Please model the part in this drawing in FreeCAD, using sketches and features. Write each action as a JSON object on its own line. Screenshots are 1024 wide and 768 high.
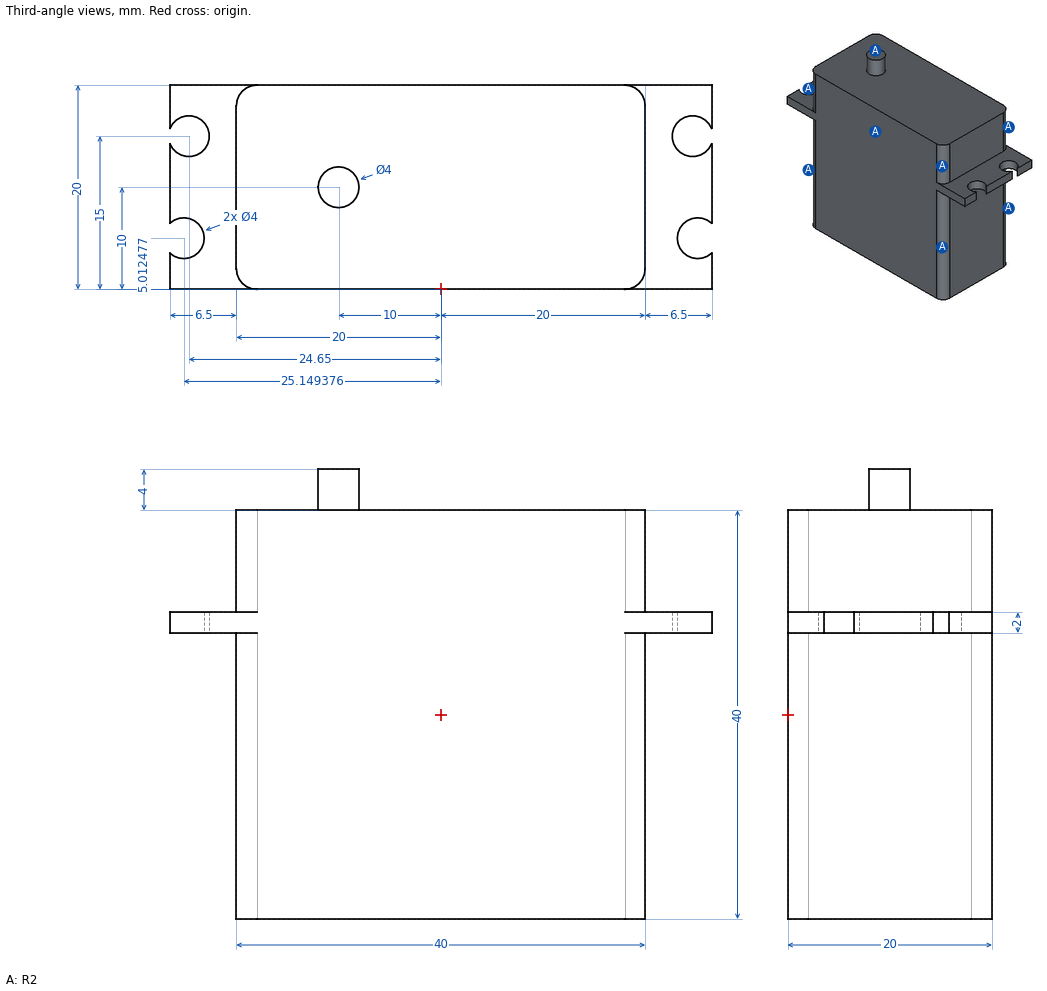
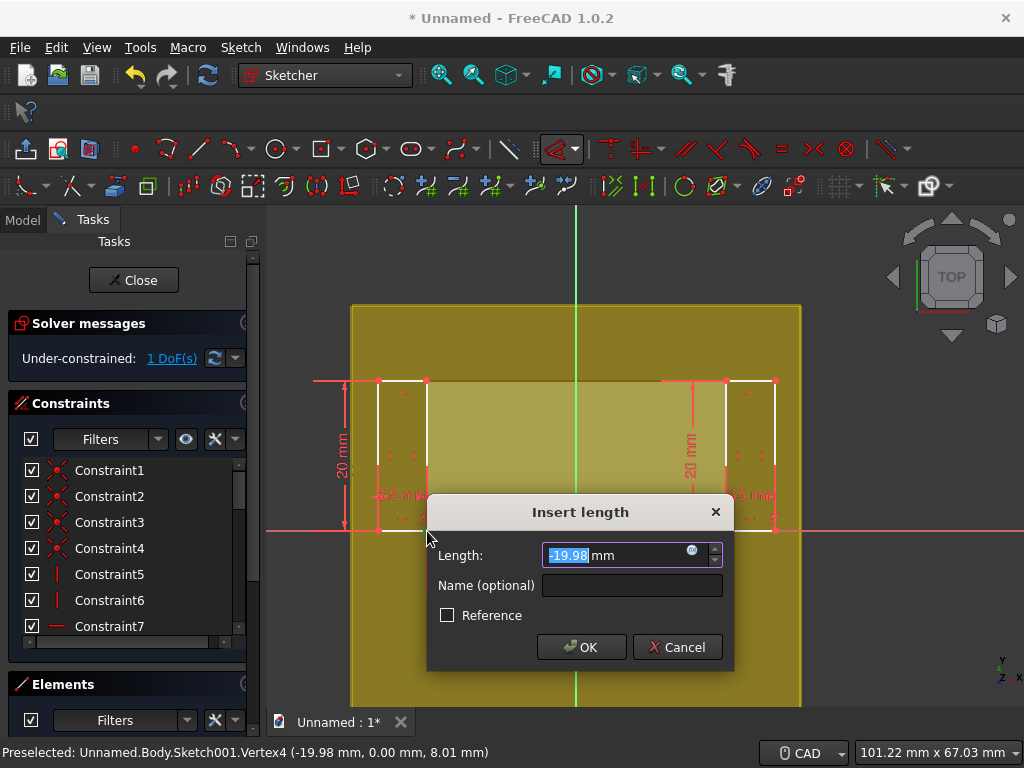
{"action": "type", "text": "-20"}
{"action": "key", "text": "Return"}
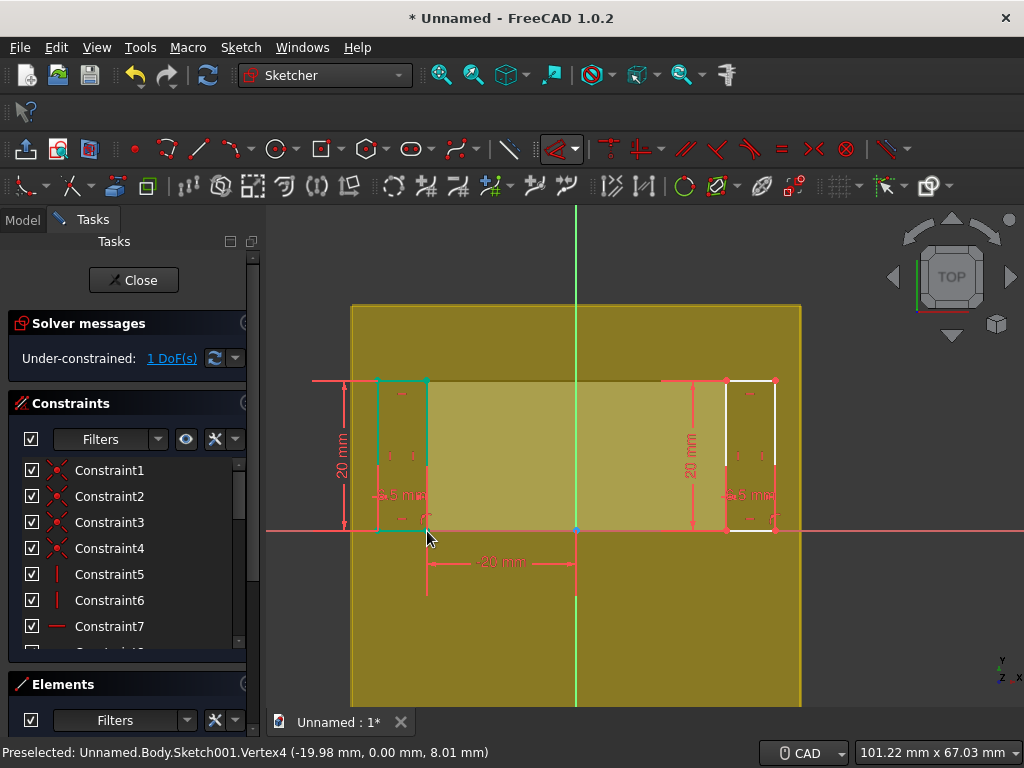
{"action": "left_click", "coordinate": [726, 381]}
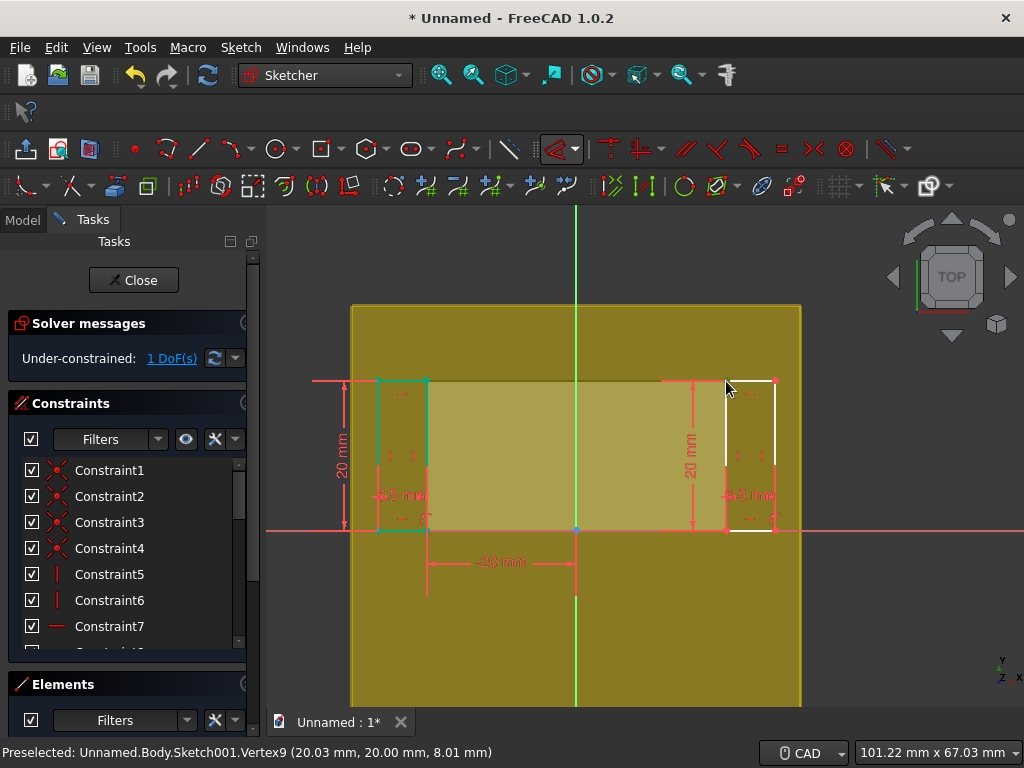
{"action": "key", "text": "l"}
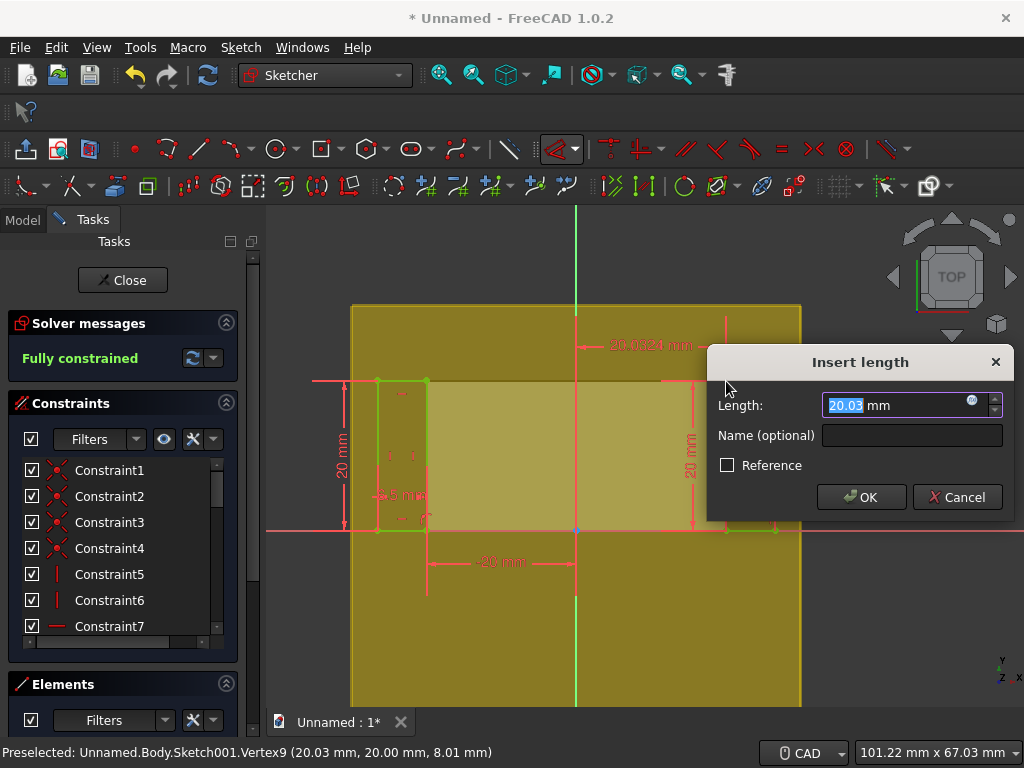
{"action": "type", "text": "20"}
{"action": "key", "text": "Return"}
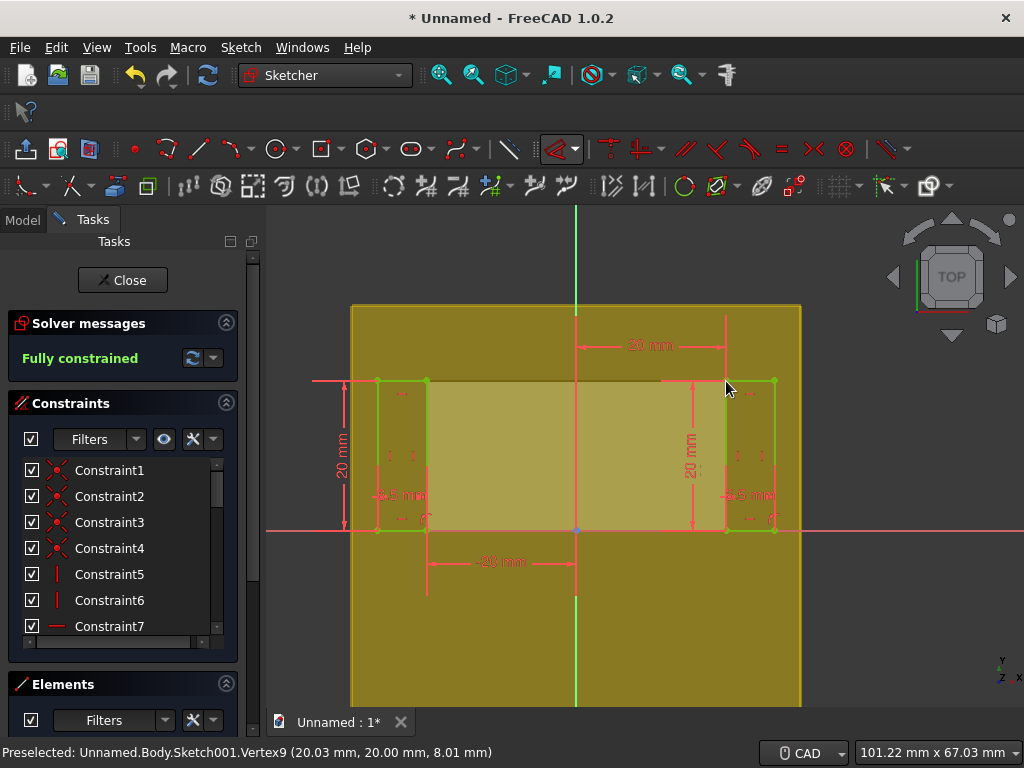
{"action": "left_click", "coordinate": [123, 280]}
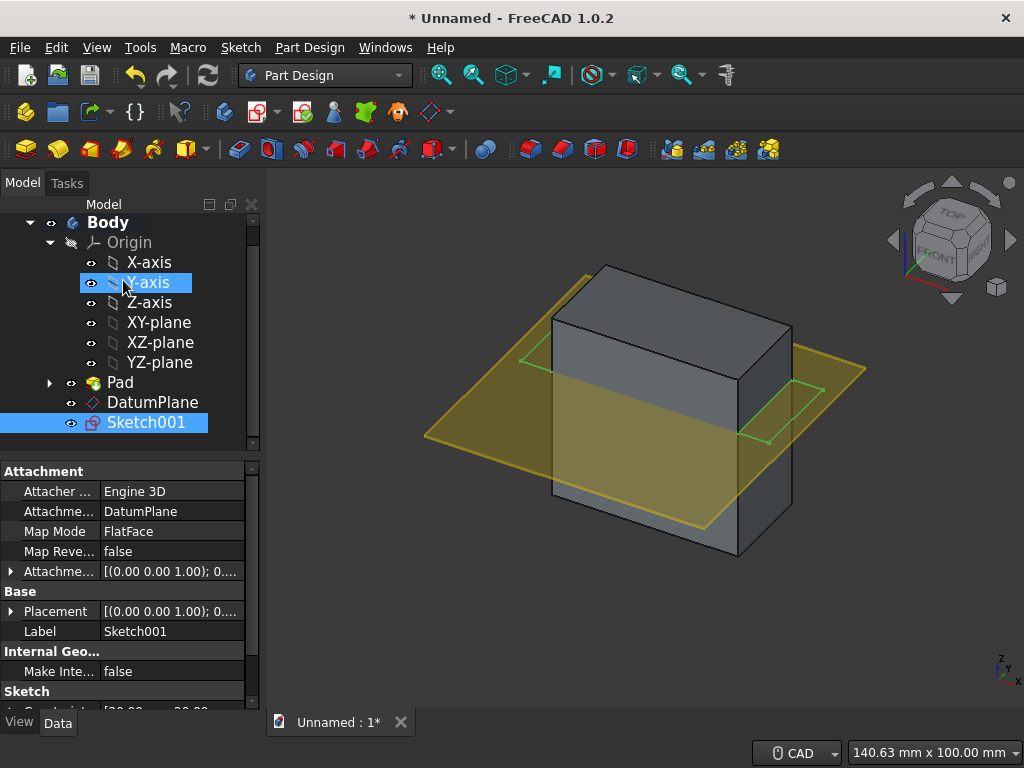
{"action": "left_click", "coordinate": [26, 150]}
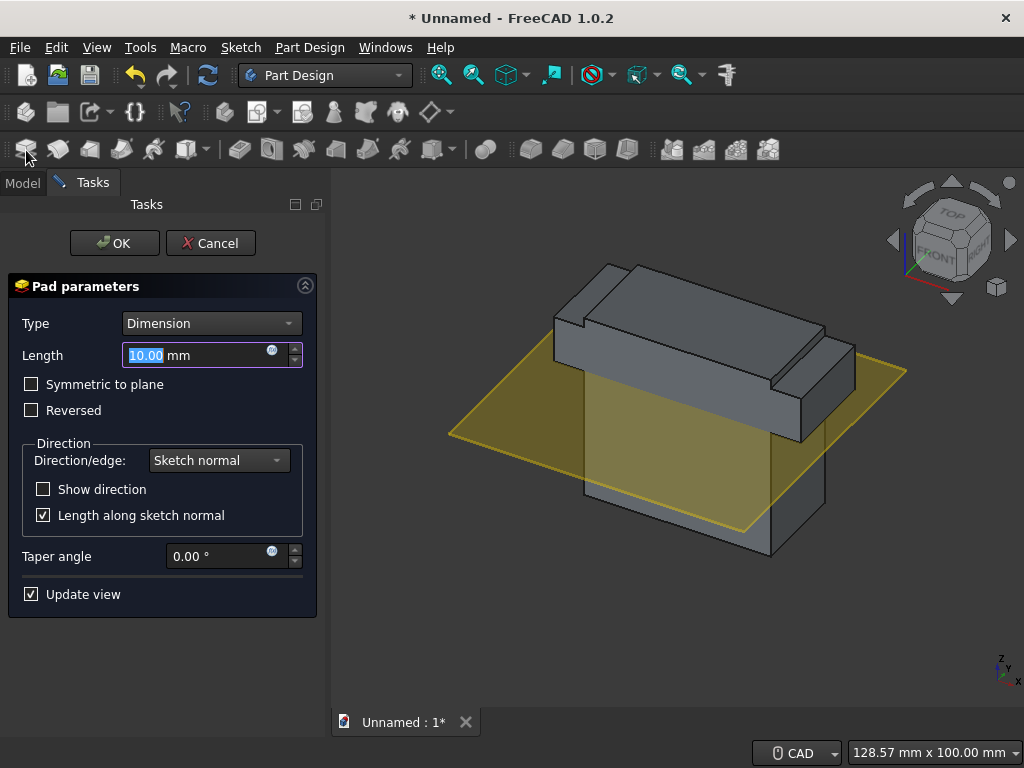
{"action": "type", "text": "2"}
{"action": "key", "text": "Tab"}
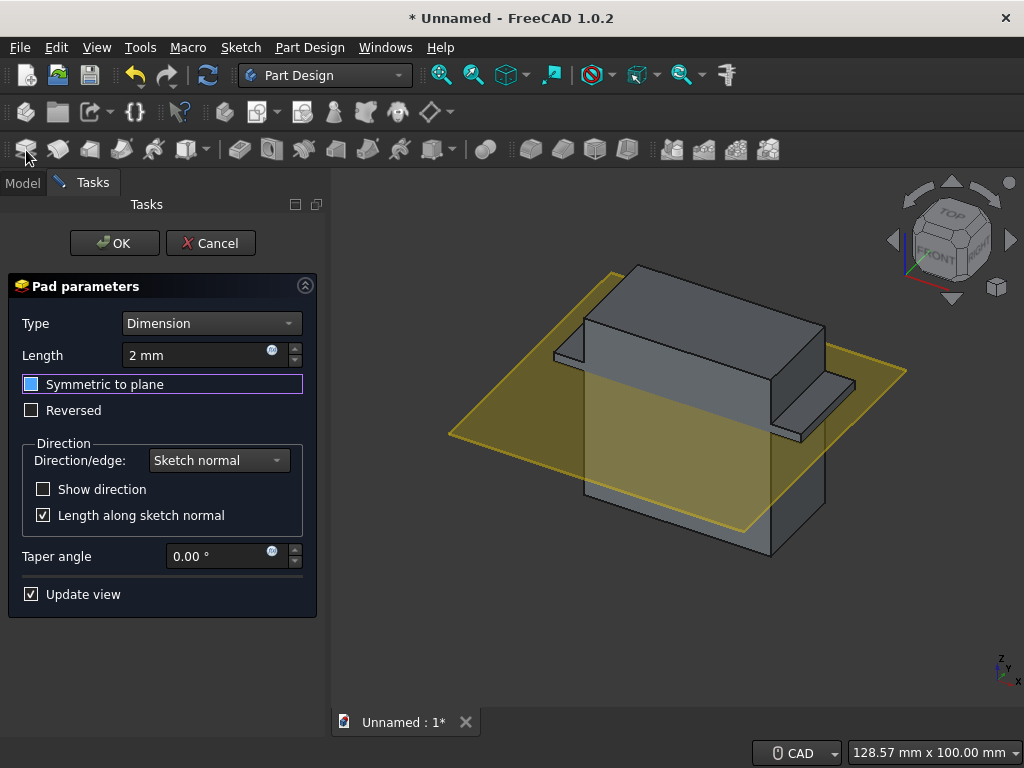
{"action": "left_click", "coordinate": [115, 243]}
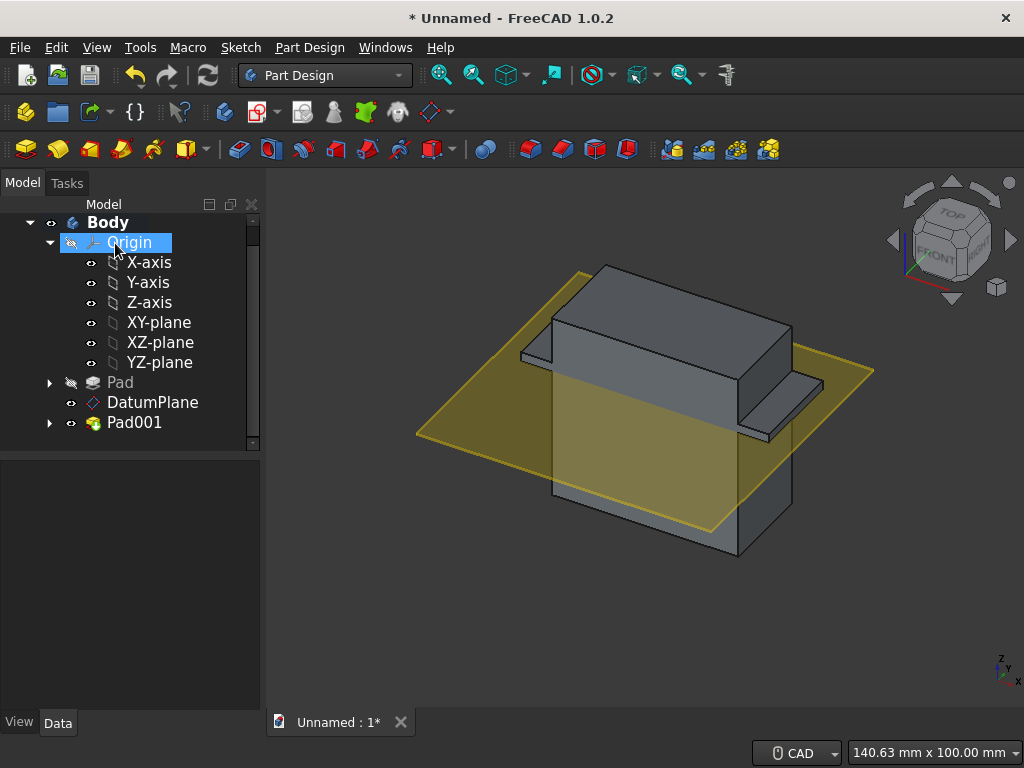
{"action": "left_click", "coordinate": [116, 403]}
{"action": "key", "text": "space"}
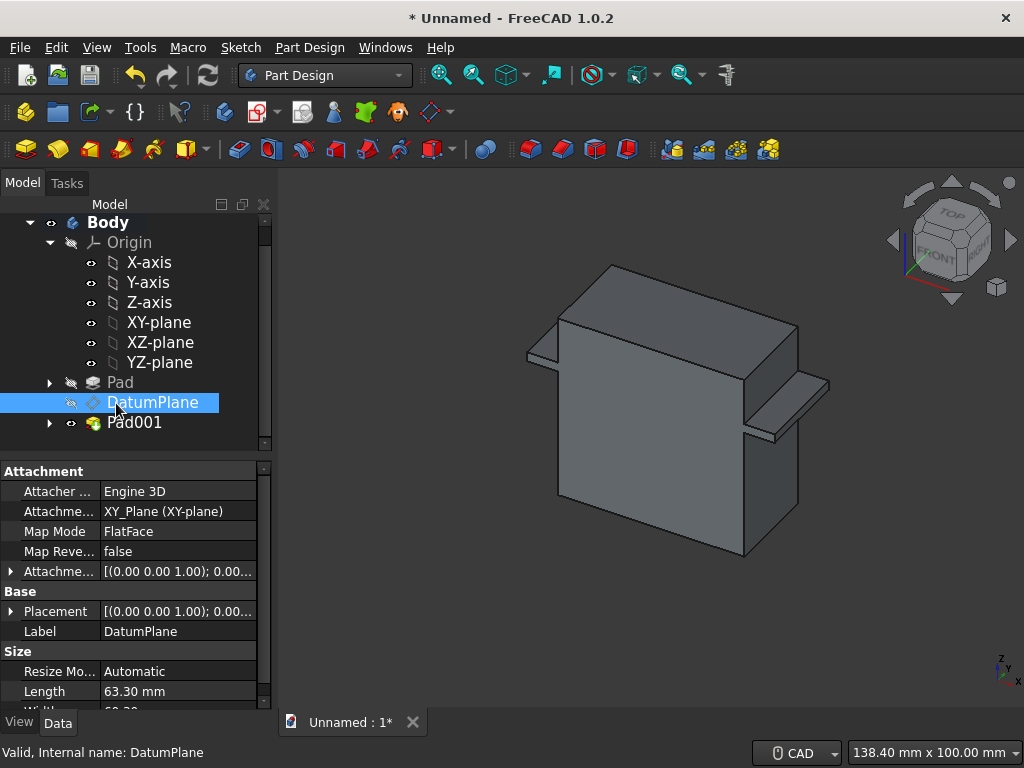
{"action": "key", "text": "5"}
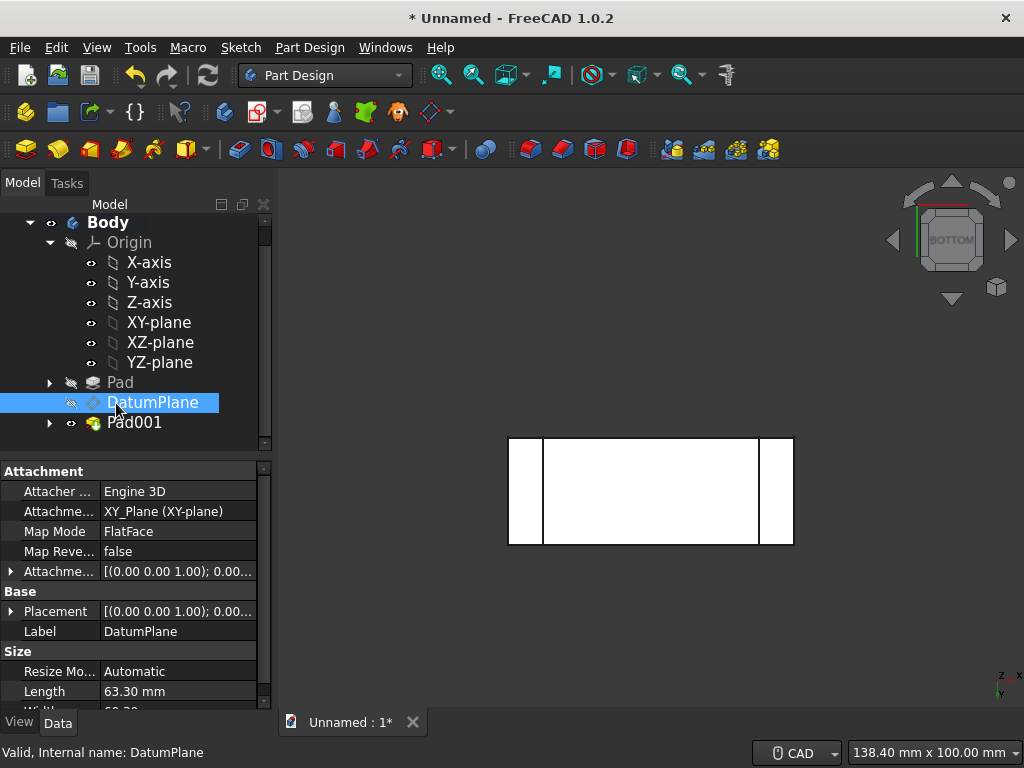
{"action": "left_click", "coordinate": [442, 76]}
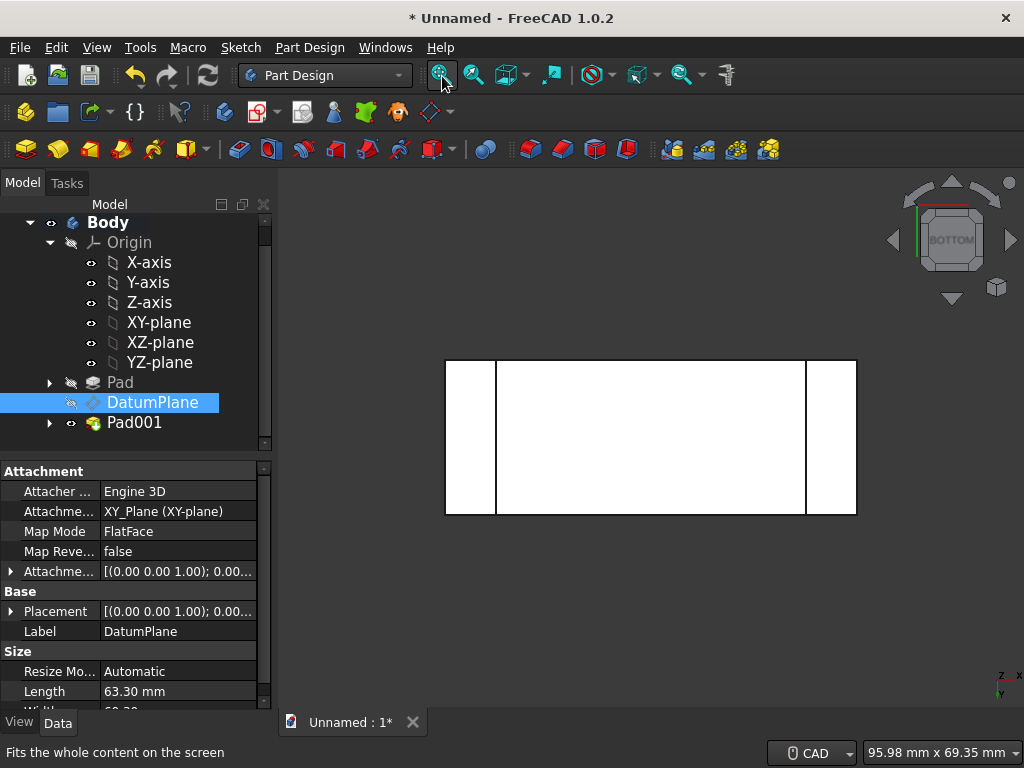
{"action": "left_click", "coordinate": [832, 481]}